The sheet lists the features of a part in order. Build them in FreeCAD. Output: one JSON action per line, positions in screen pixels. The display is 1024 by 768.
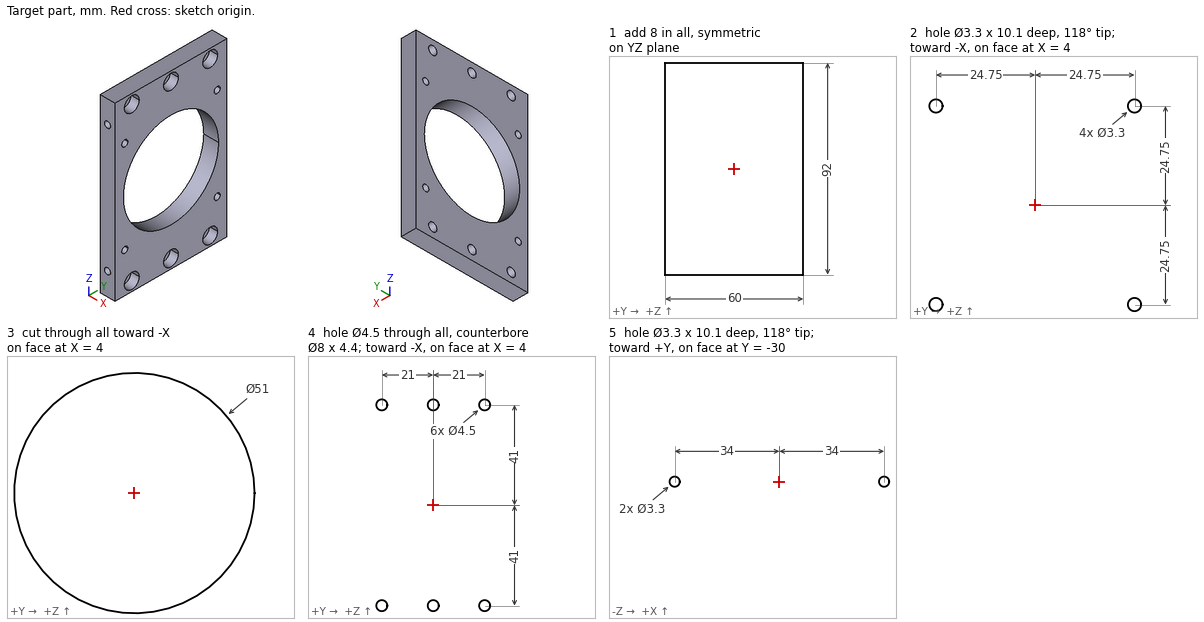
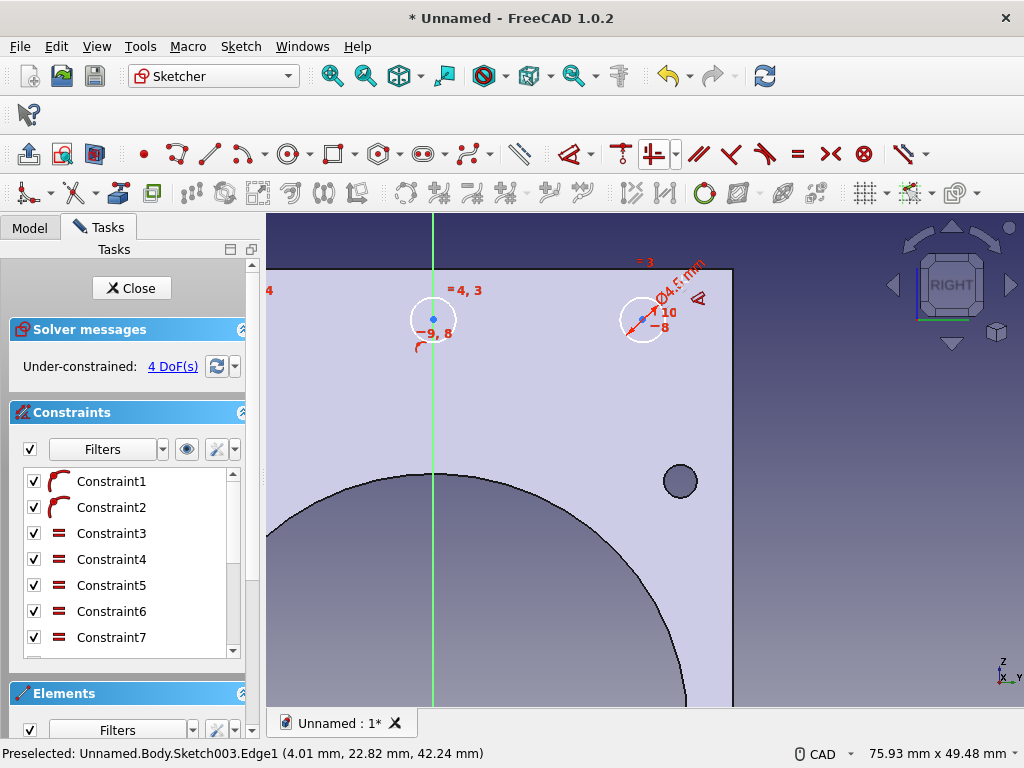
{"action": "left_click", "coordinate": [643, 320]}
{"action": "left_click", "coordinate": [538, 286]}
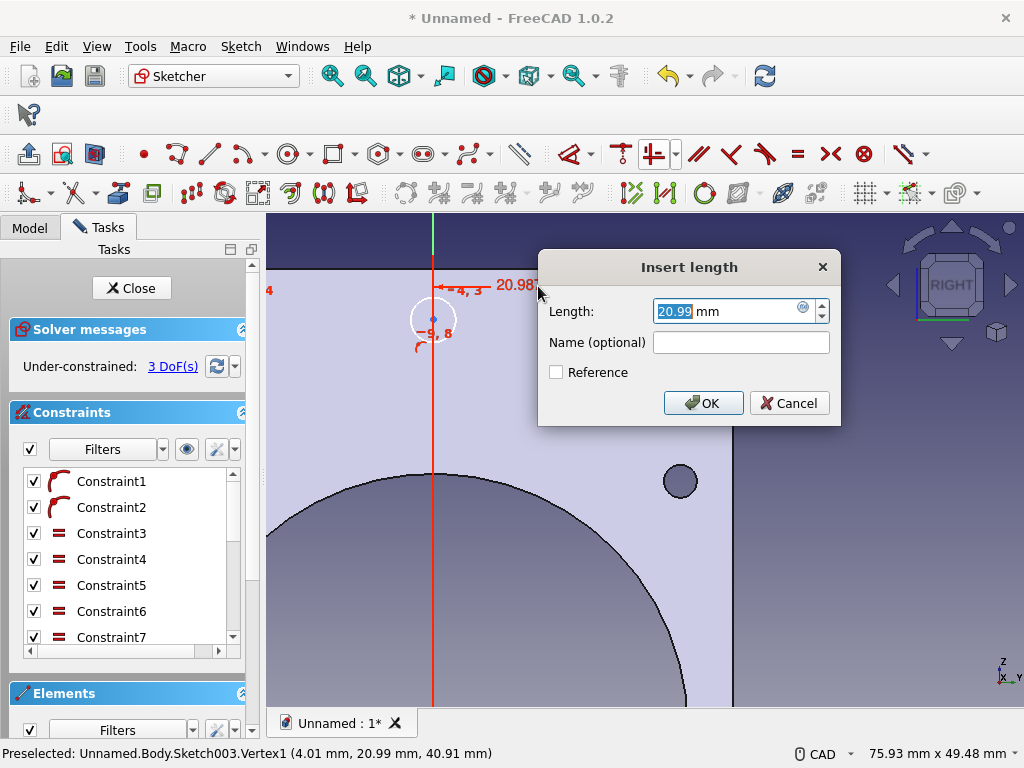
{"action": "type", "text": "21"}
{"action": "key", "text": "Return"}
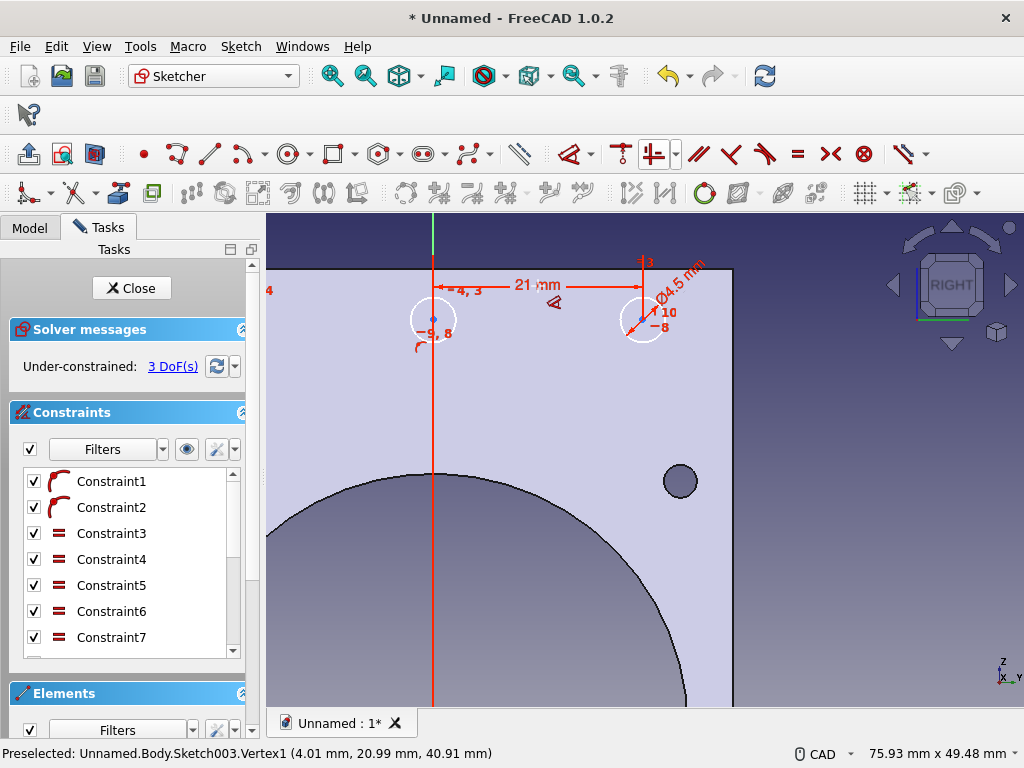
{"action": "left_click", "coordinate": [643, 320]}
{"action": "left_click", "coordinate": [677, 499]}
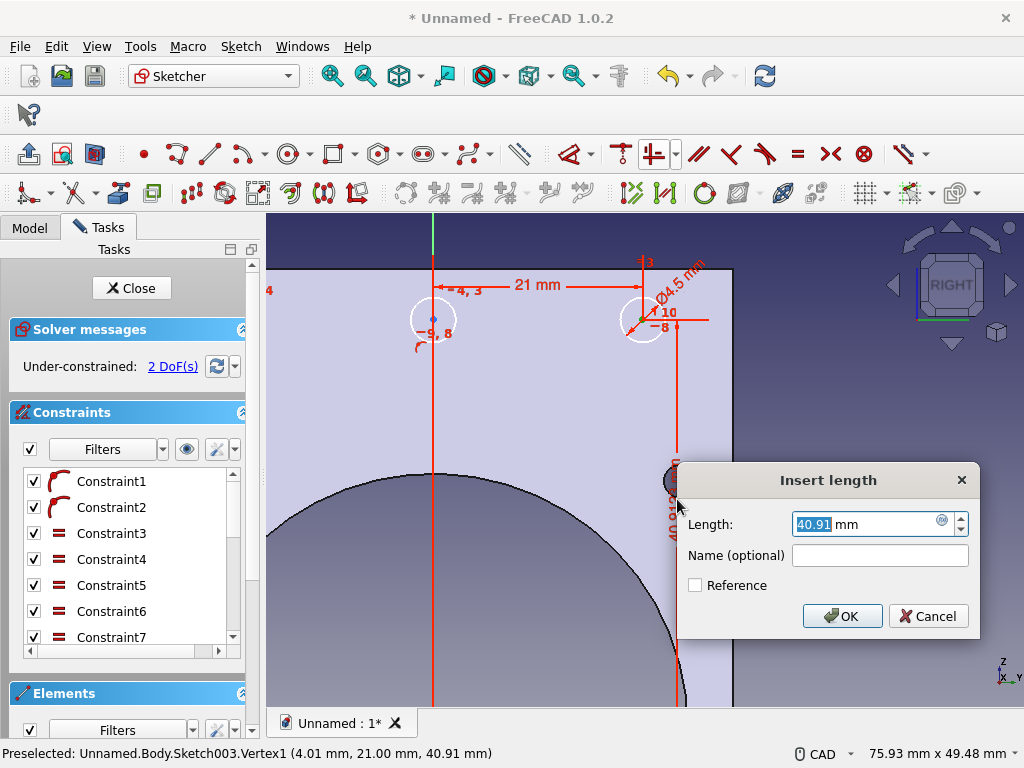
{"action": "type", "text": "41"}
{"action": "key", "text": "Return"}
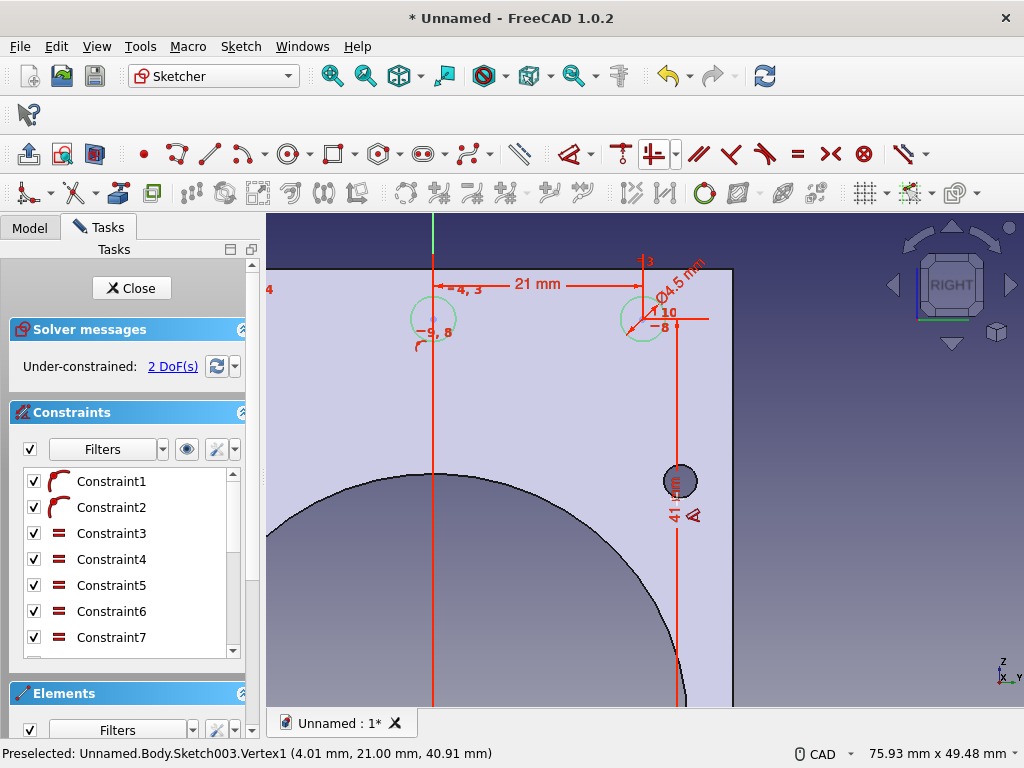
{"action": "scroll", "coordinate": [660, 304], "scroll_direction": "down", "scroll_amount": 5}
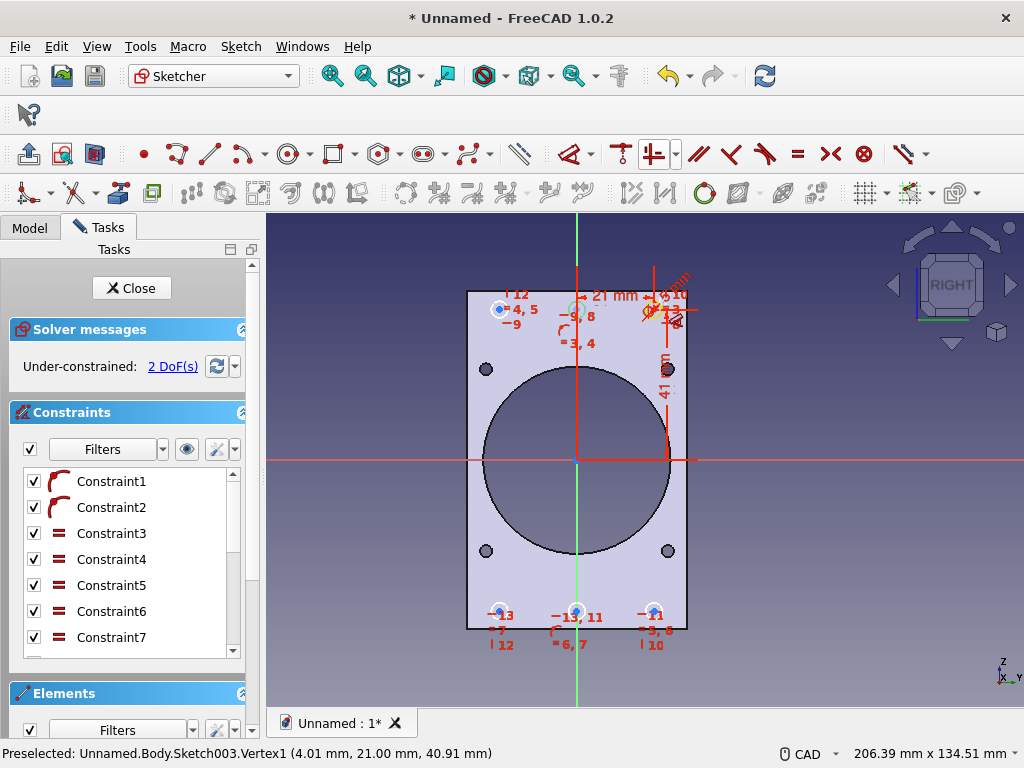
{"action": "left_click", "coordinate": [500, 310]}
{"action": "left_click", "coordinate": [538, 276]}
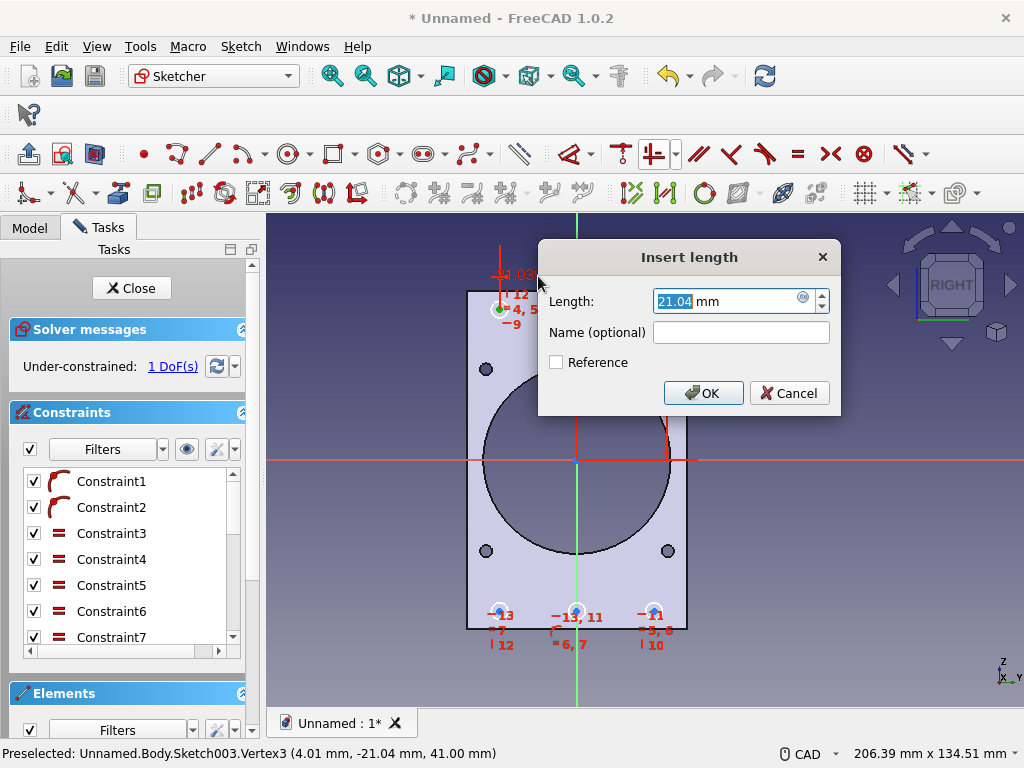
{"action": "type", "text": "21"}
{"action": "key", "text": "Return"}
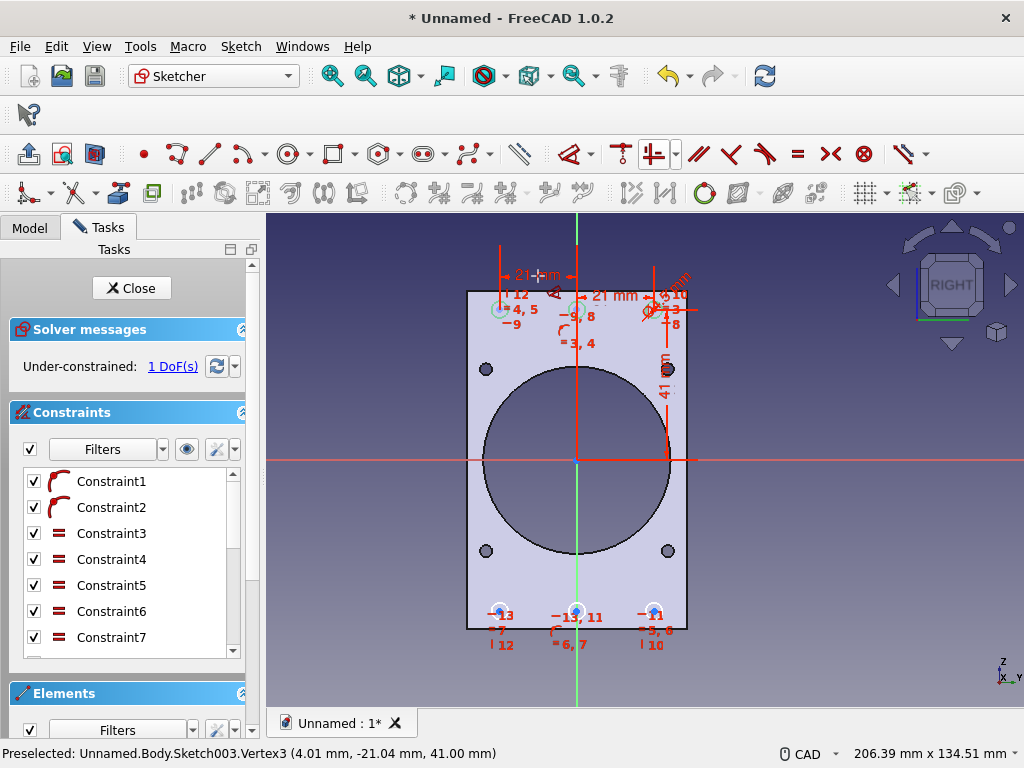
{"action": "left_click", "coordinate": [654, 611]}
{"action": "left_click", "coordinate": [688, 536]}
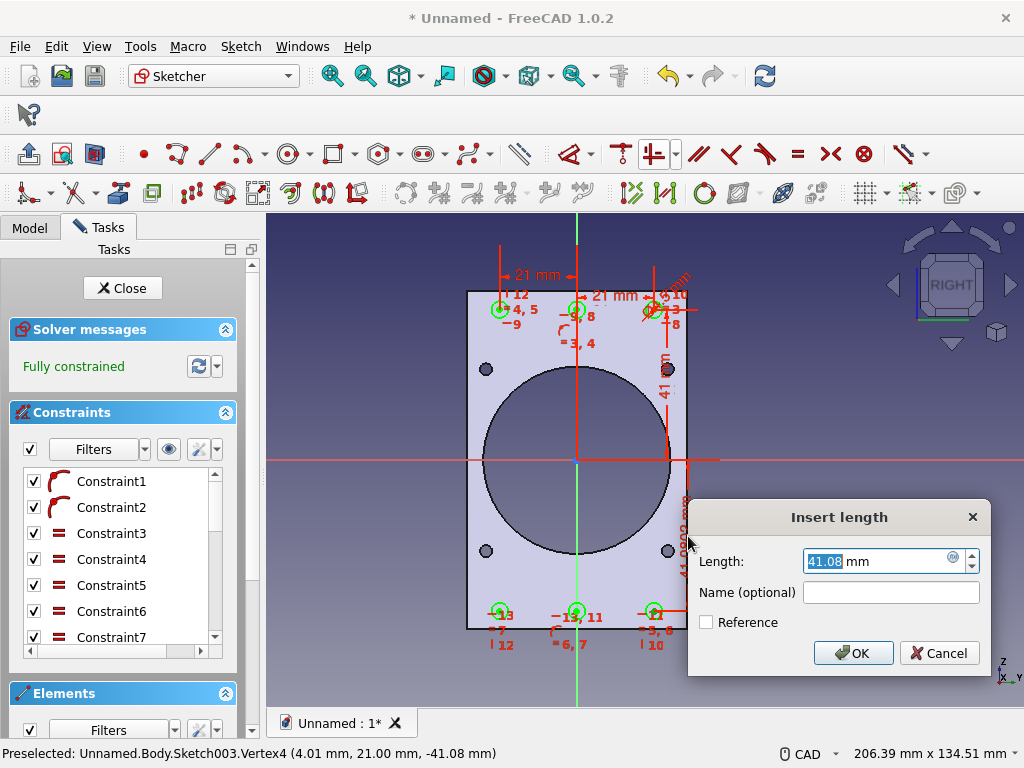
{"action": "type", "text": "41"}
{"action": "key", "text": "Return"}
{"action": "key", "text": "Escape"}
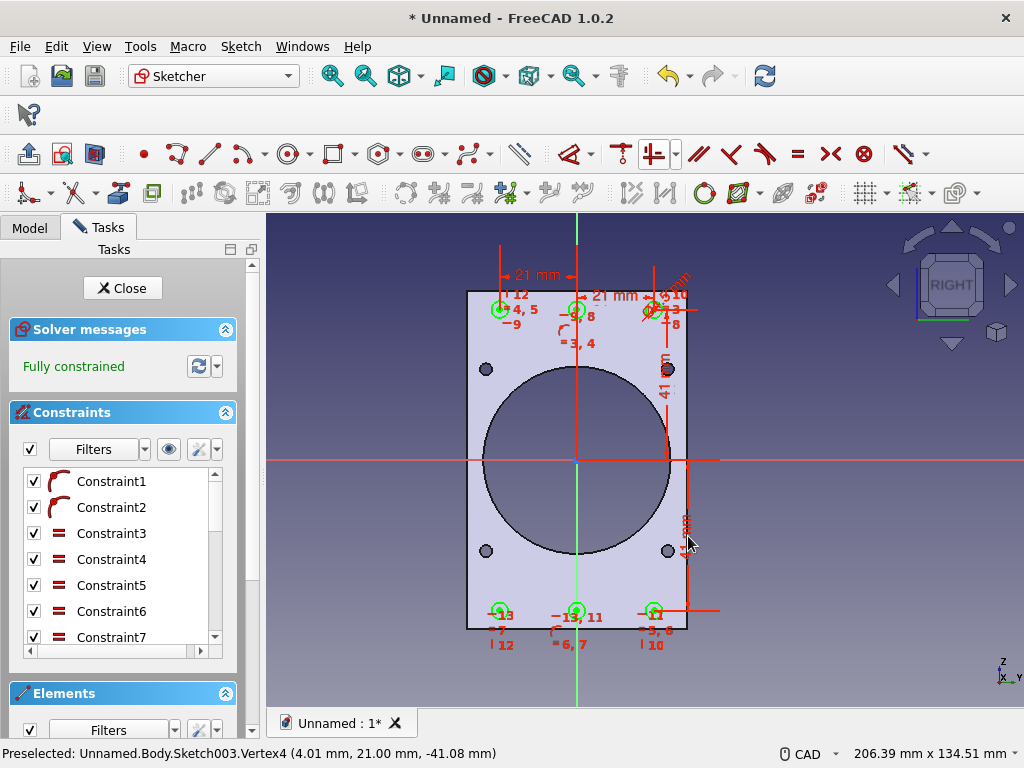
{"action": "left_click", "coordinate": [123, 288]}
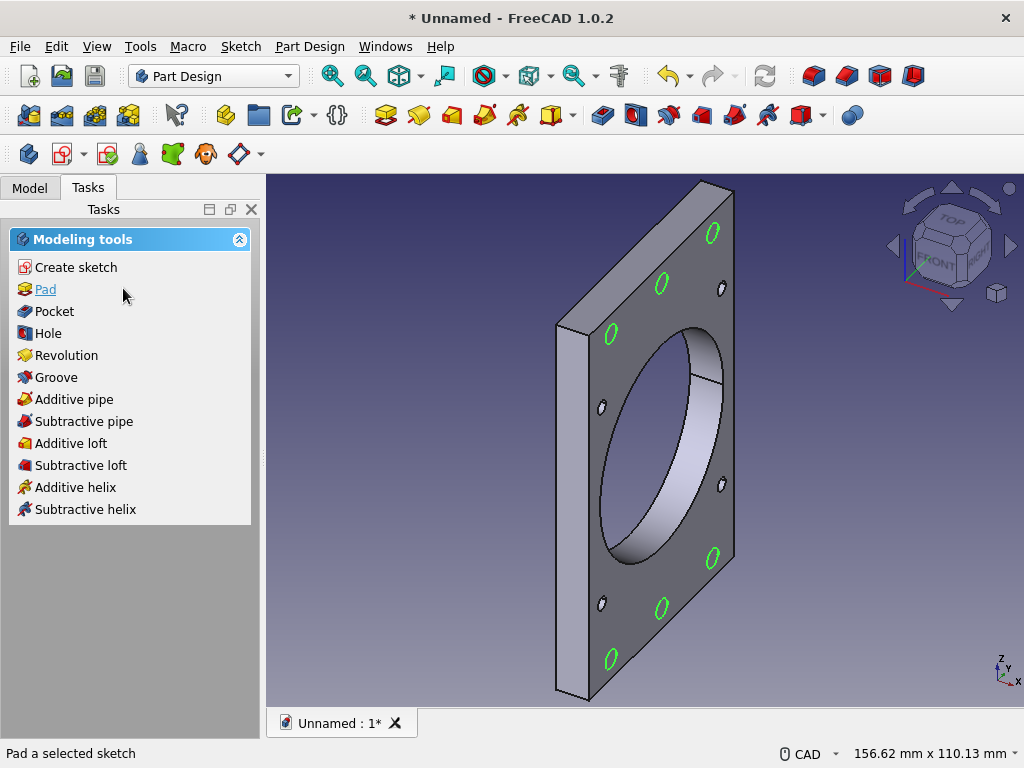
{"action": "left_click", "coordinate": [636, 116]}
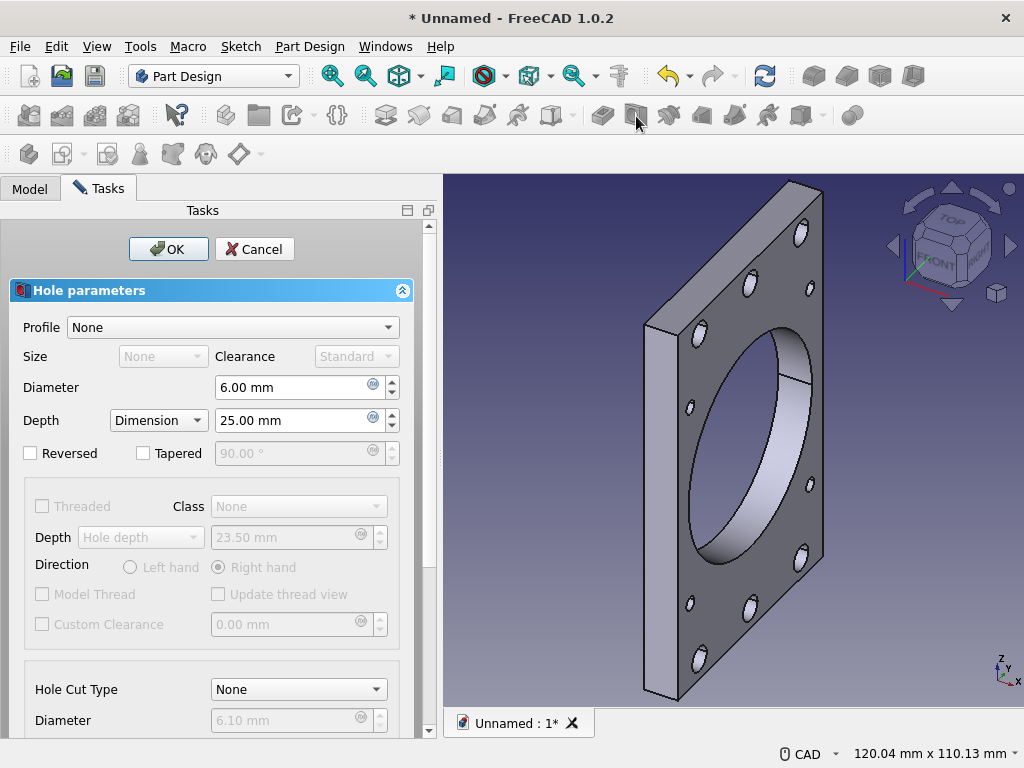
{"action": "triple_click", "coordinate": [300, 388]}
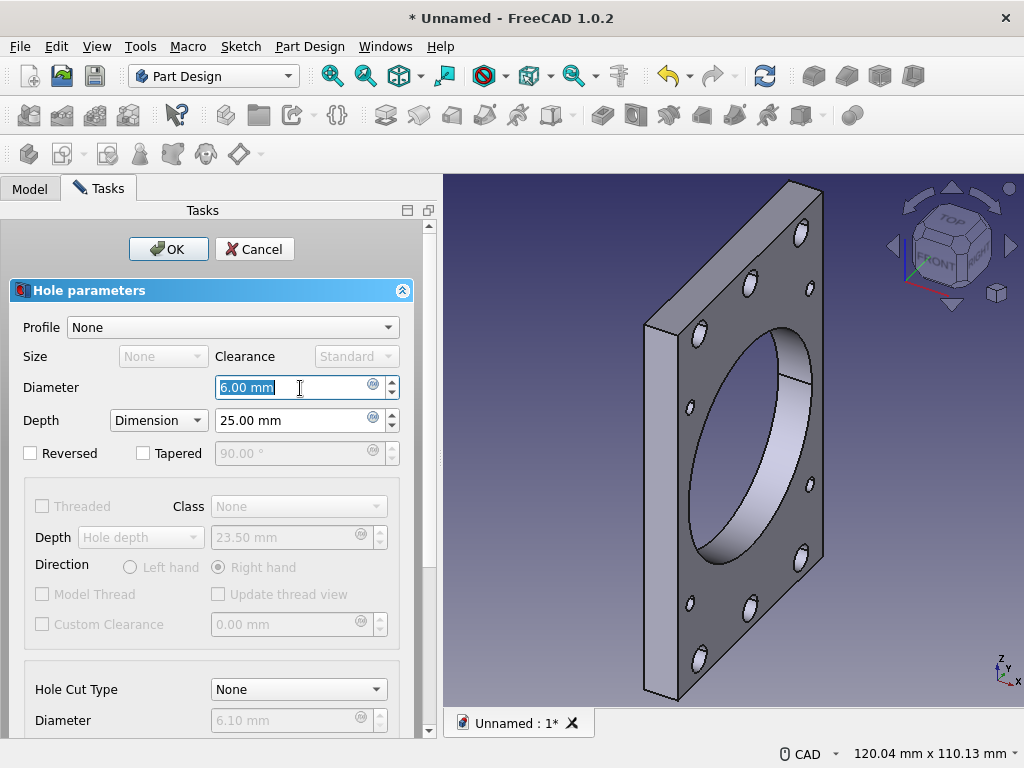
{"action": "type", "text": "4.5"}
{"action": "key", "text": "Tab"}